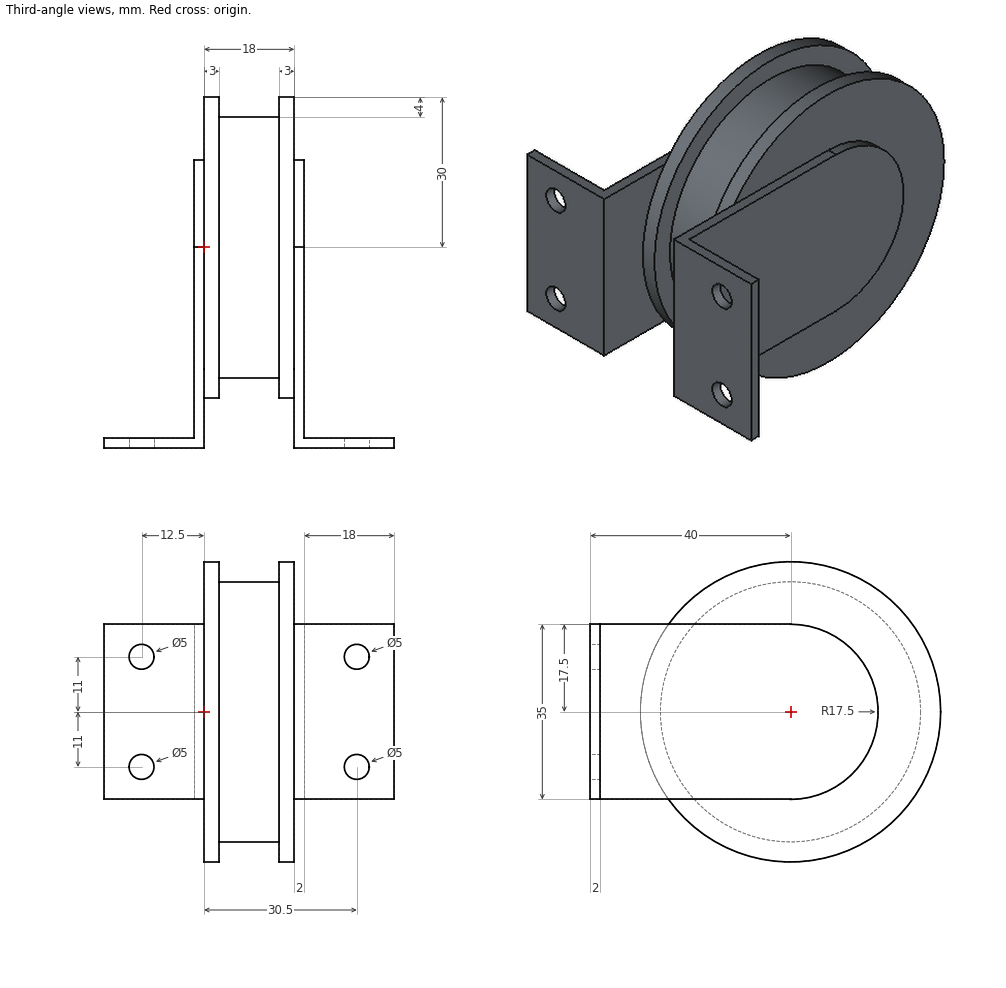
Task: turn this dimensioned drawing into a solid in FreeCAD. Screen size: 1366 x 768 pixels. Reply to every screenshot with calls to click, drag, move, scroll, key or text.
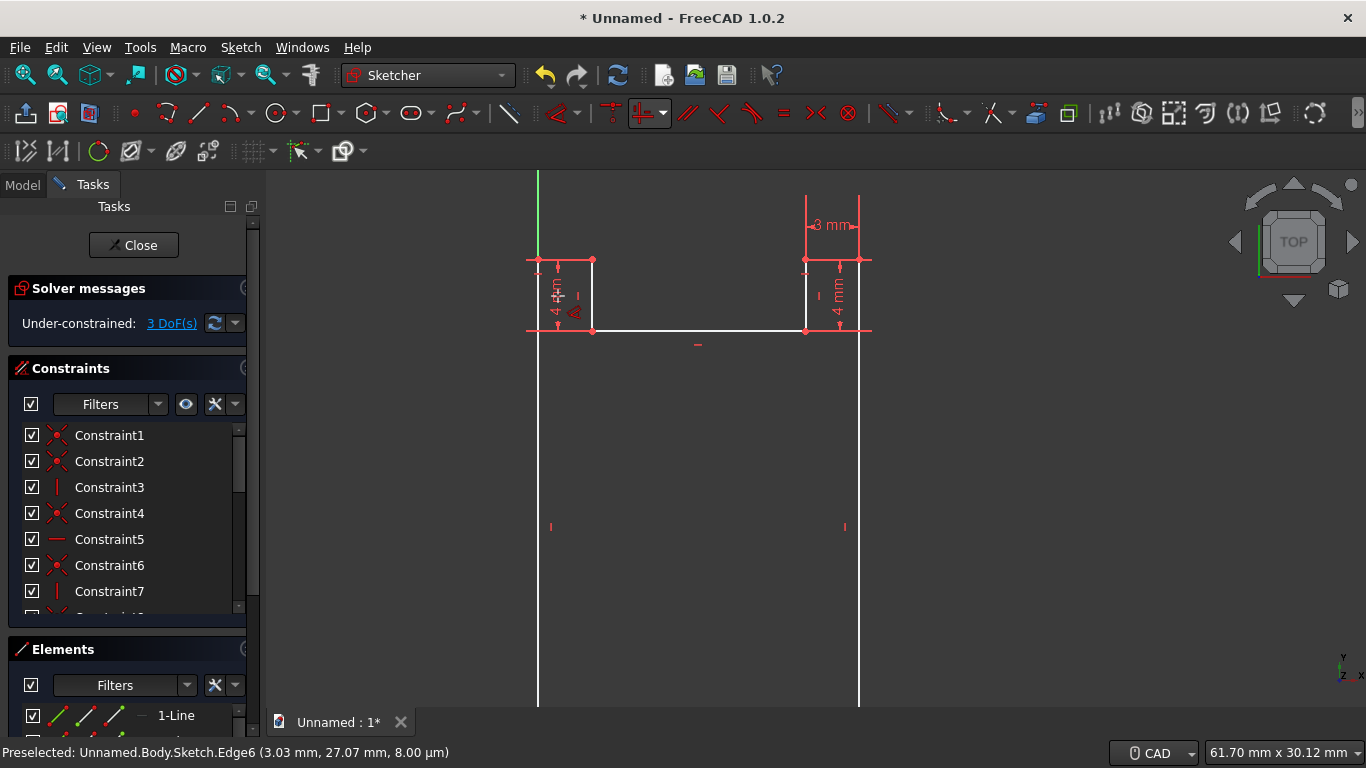
click(576, 260)
click(565, 226)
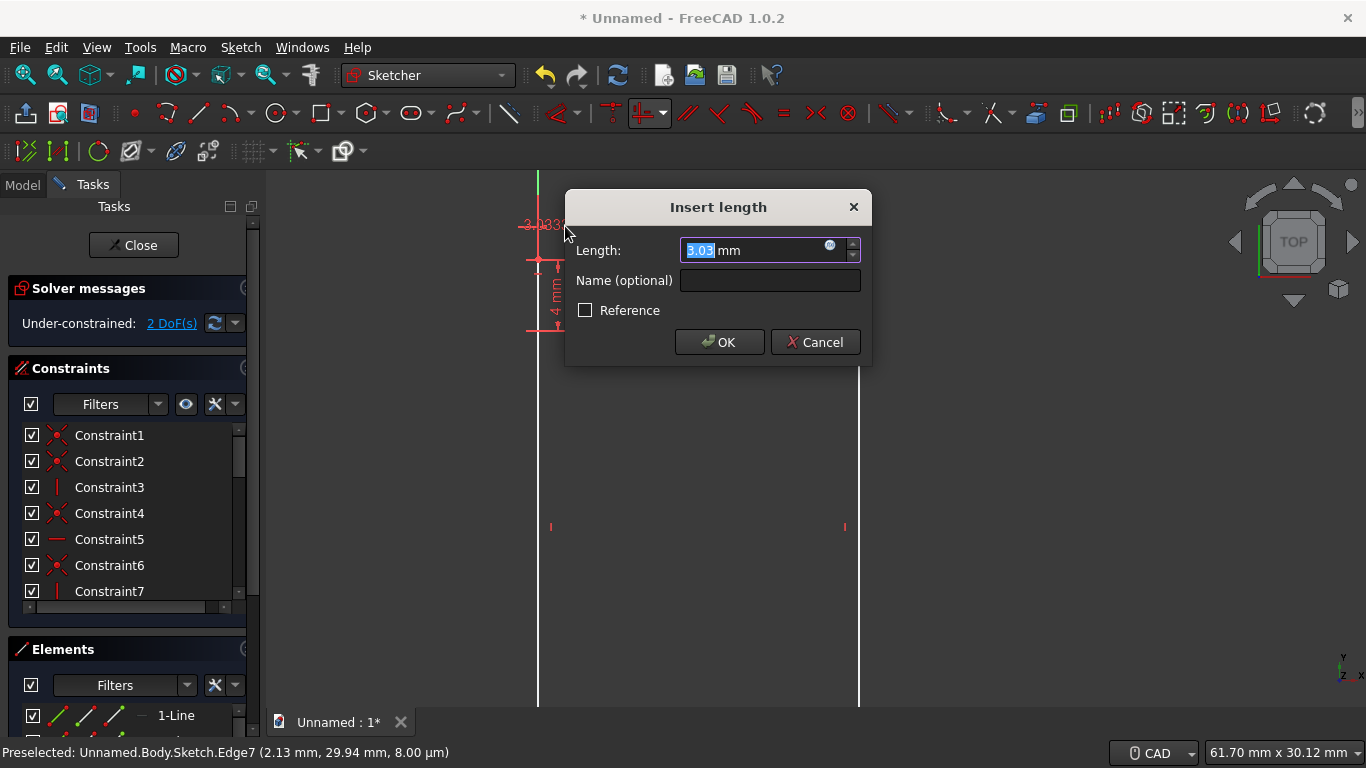
text(3)
key(Return)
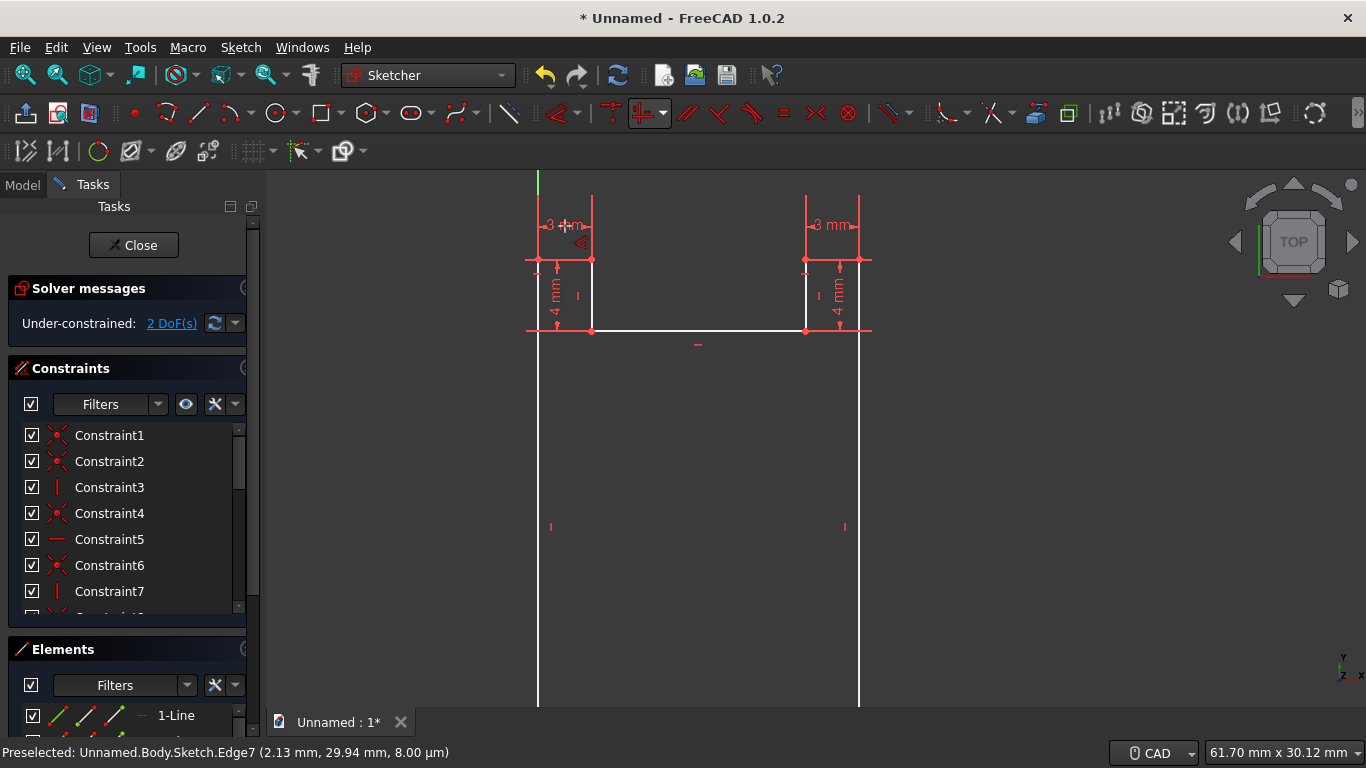
scroll(847, 260, down, 2)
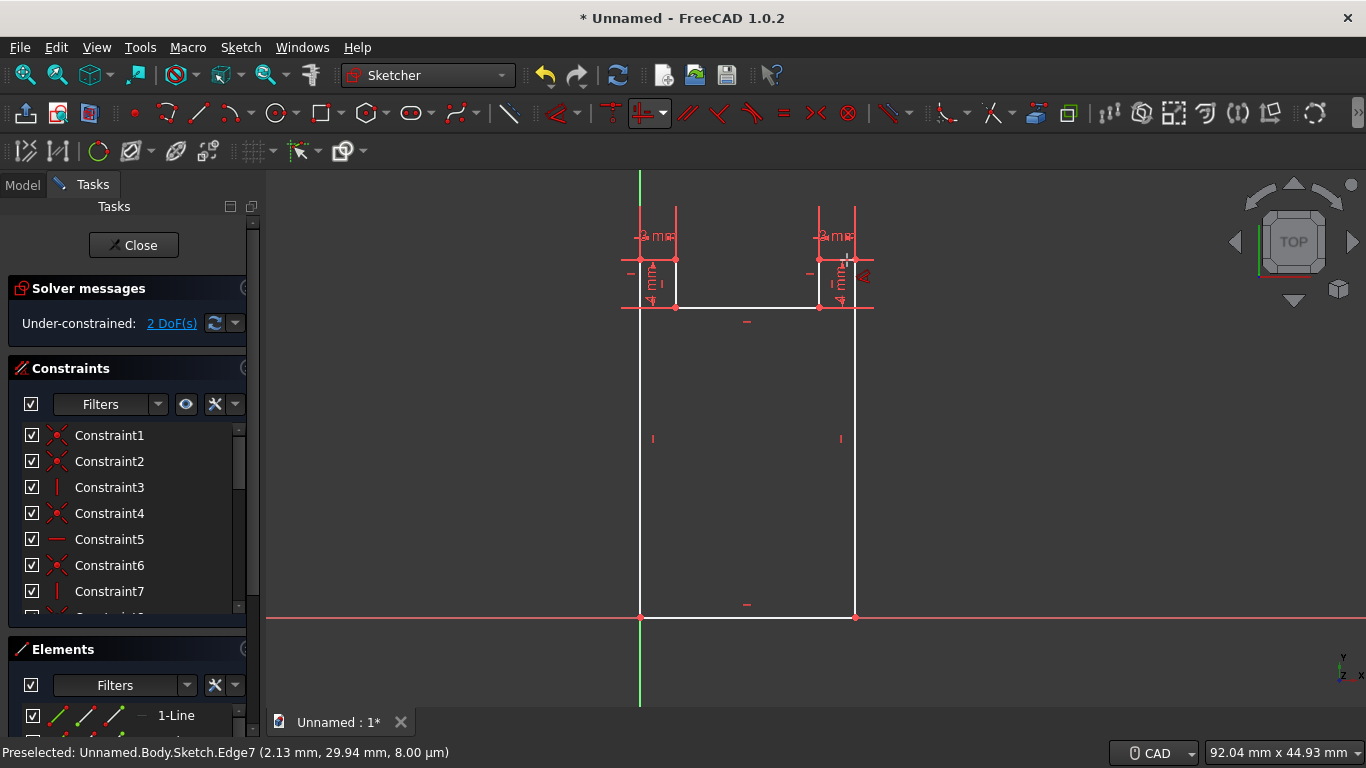
click(705, 618)
click(748, 652)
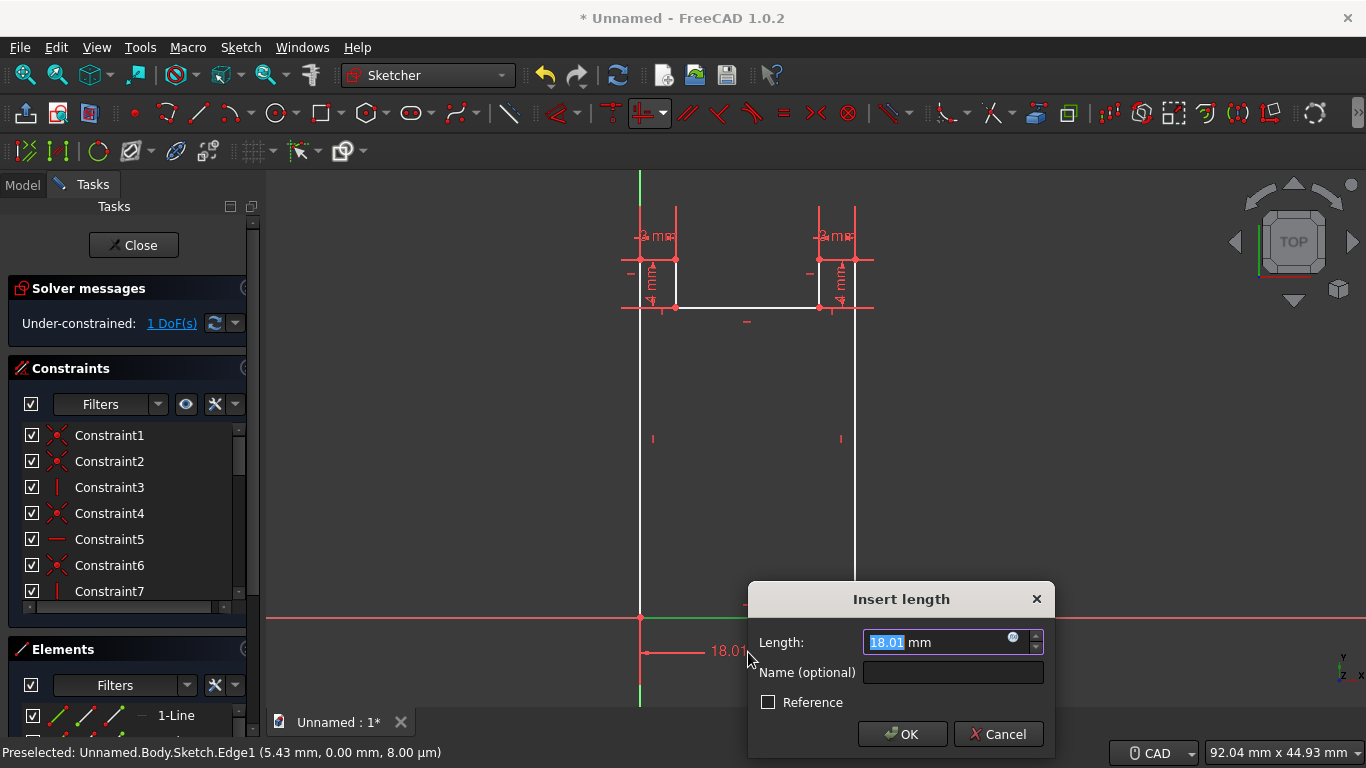
text(18)
key(Return)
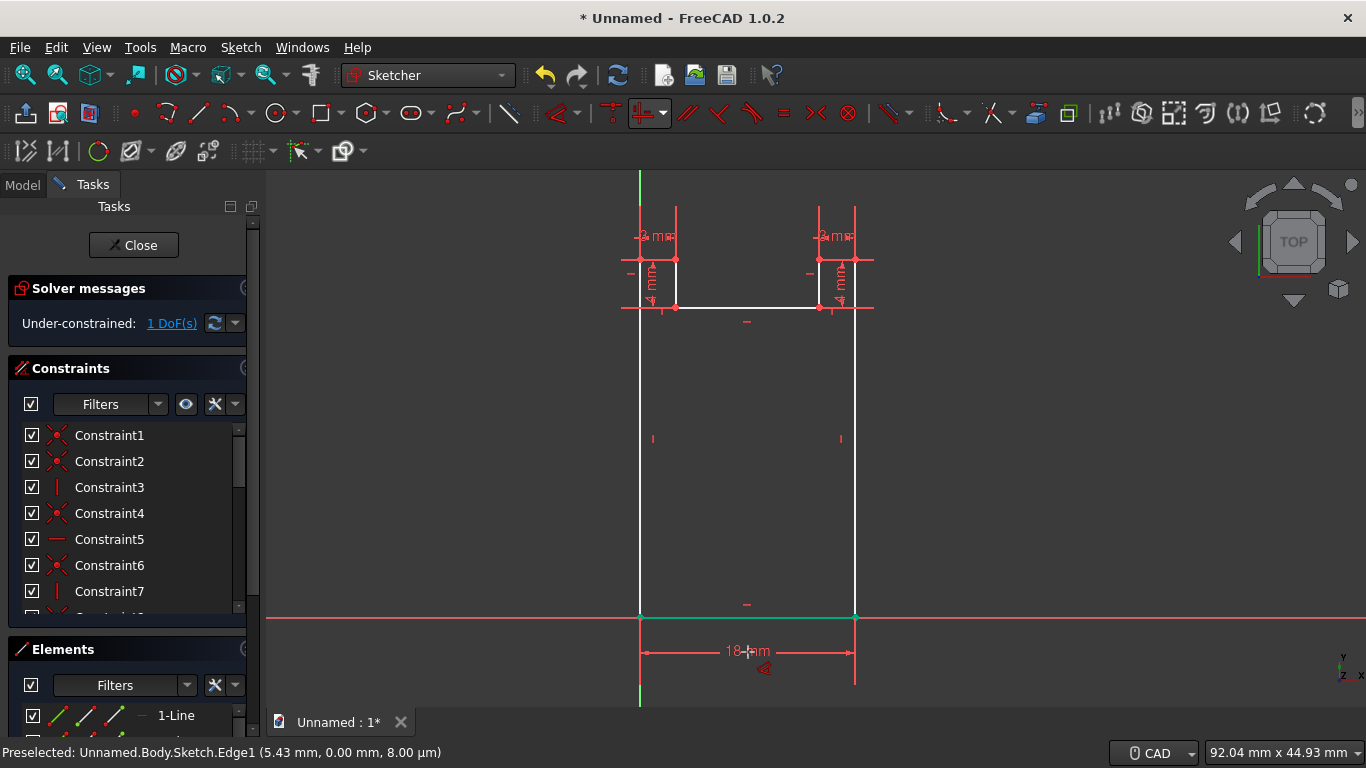
click(855, 510)
click(889, 439)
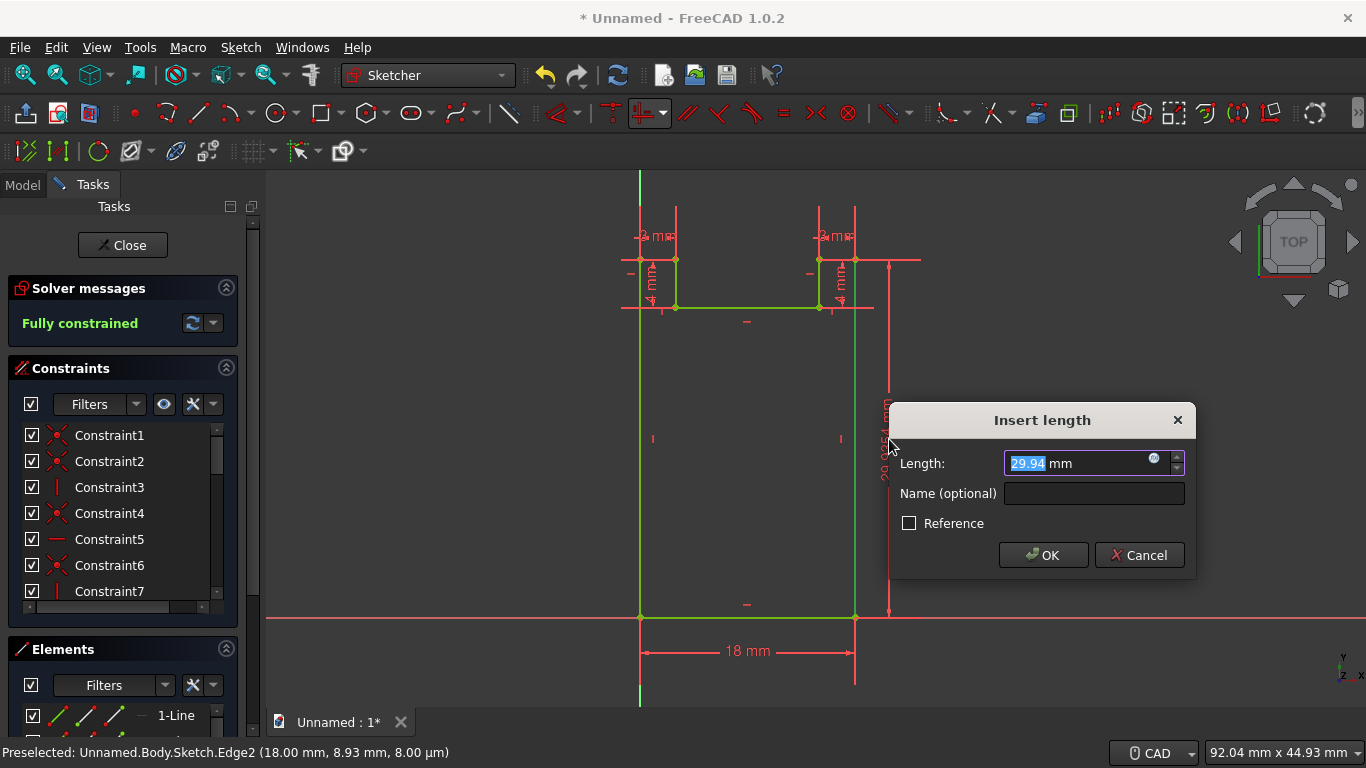
text(30)
key(Return)
key(Escape)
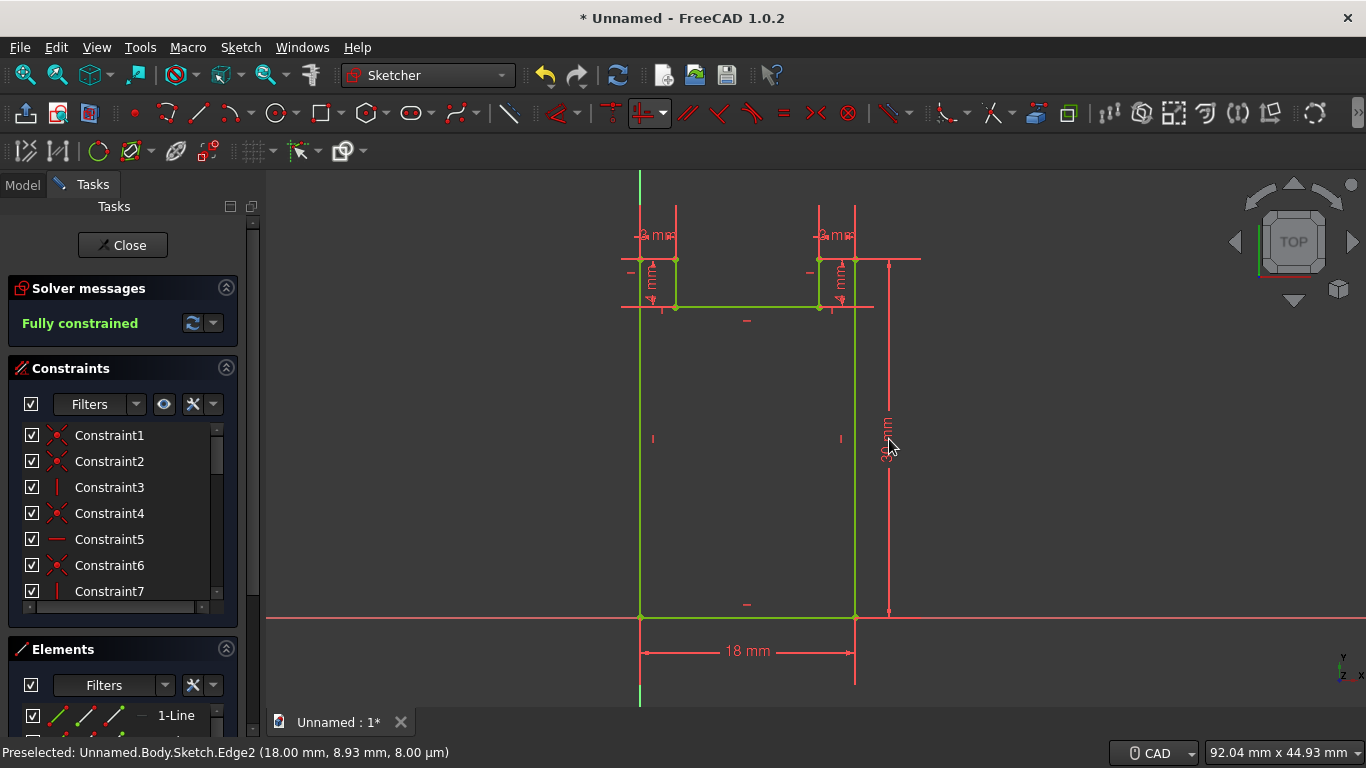
click(123, 245)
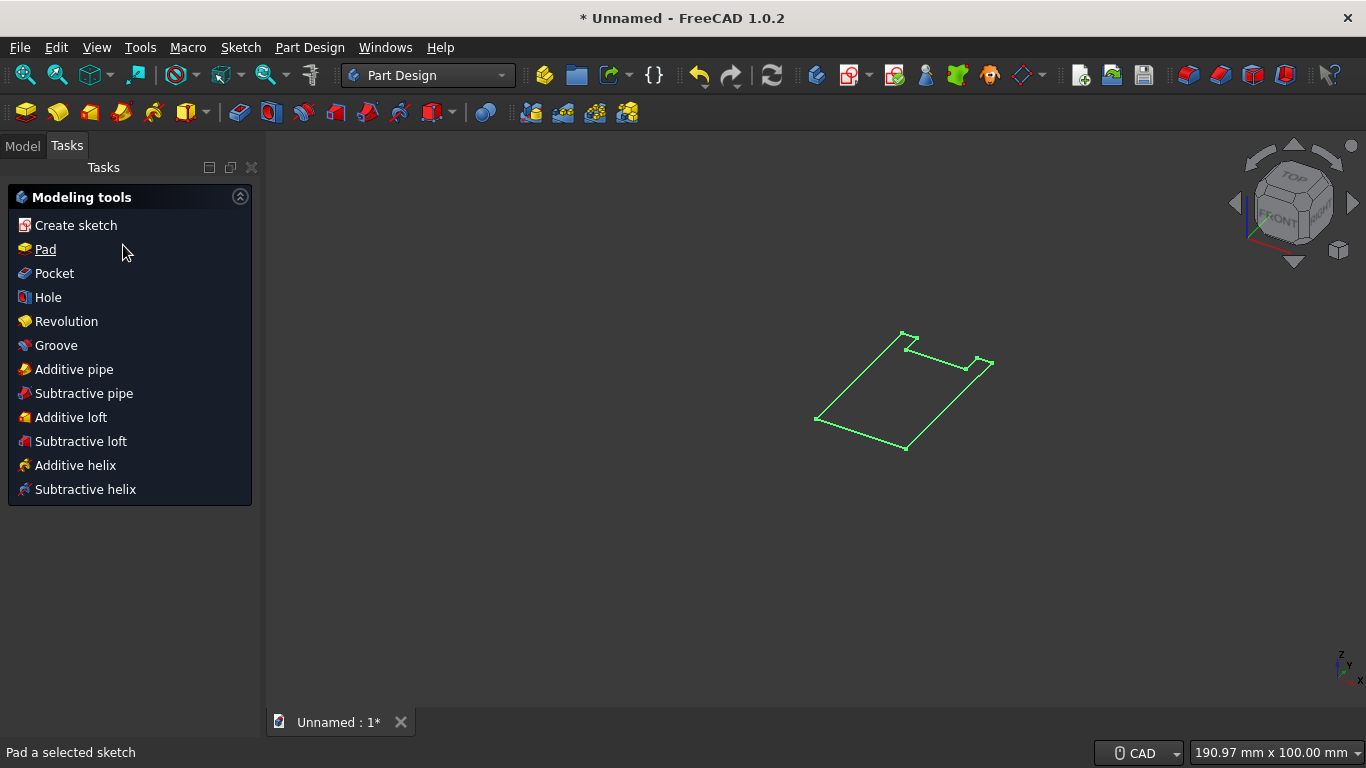
click(58, 112)